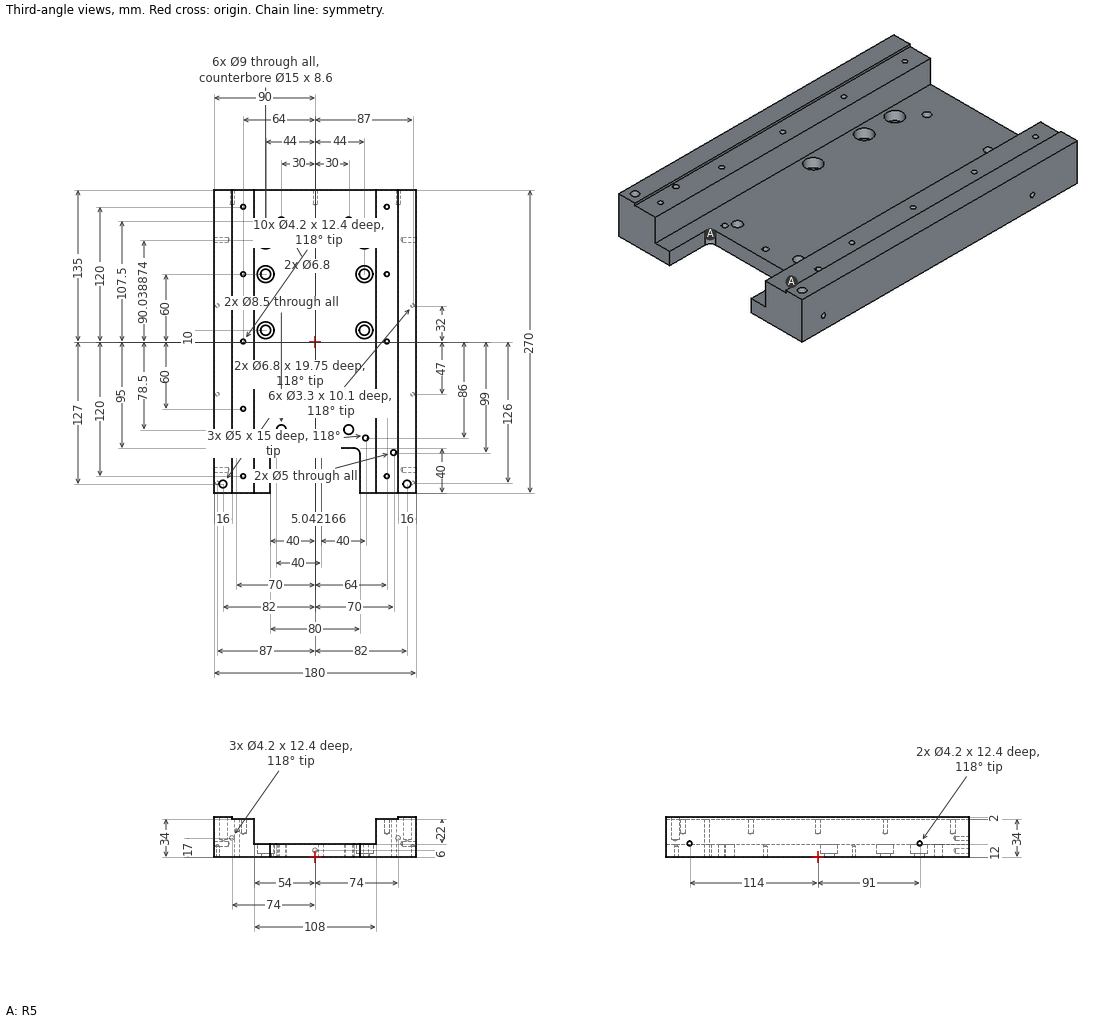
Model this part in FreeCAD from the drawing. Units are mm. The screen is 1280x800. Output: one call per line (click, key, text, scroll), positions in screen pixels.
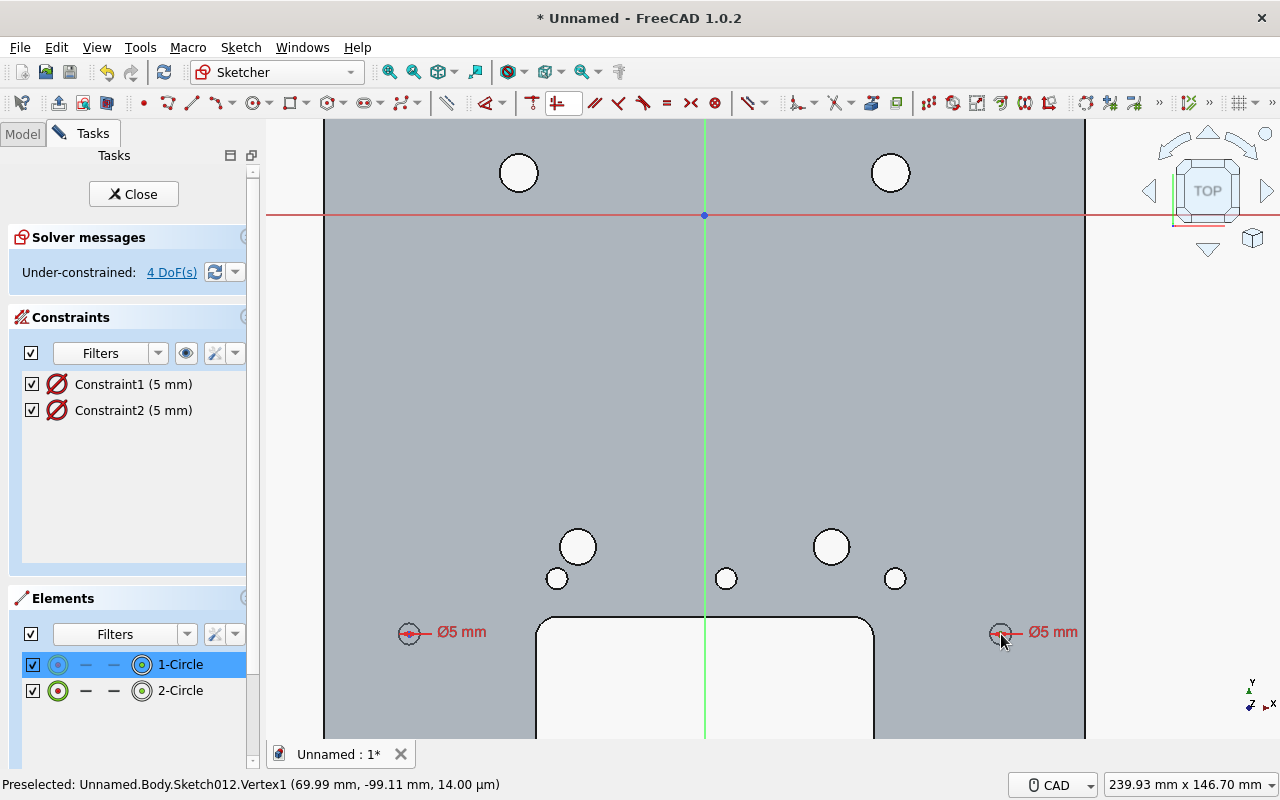
click(409, 634)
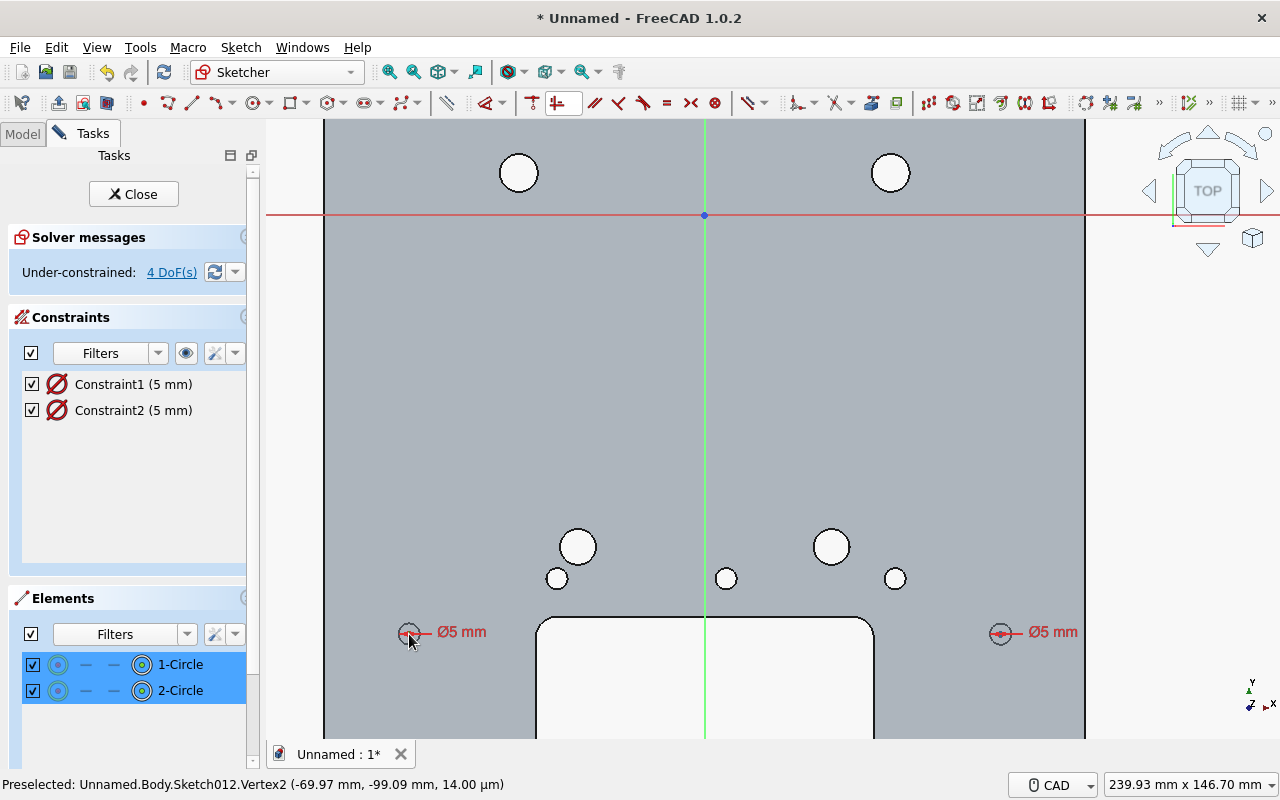
key(h)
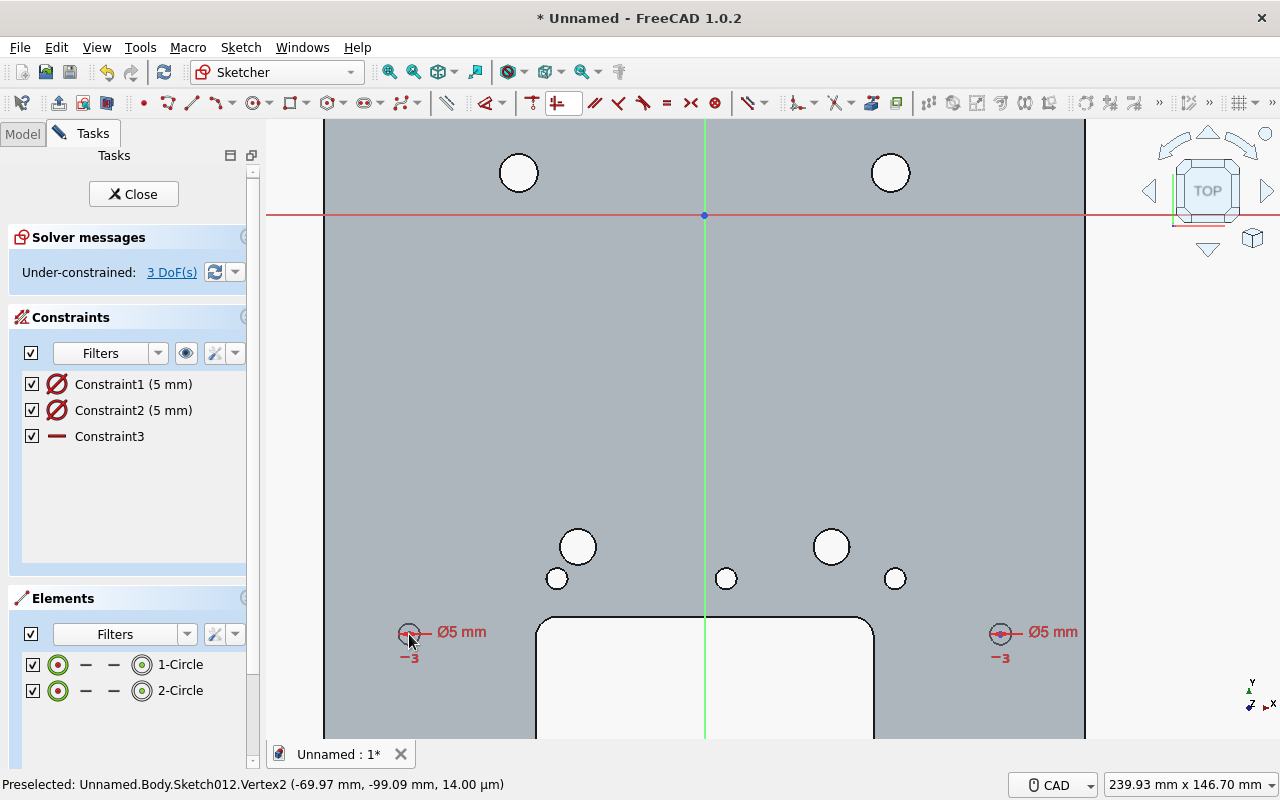
click(486, 104)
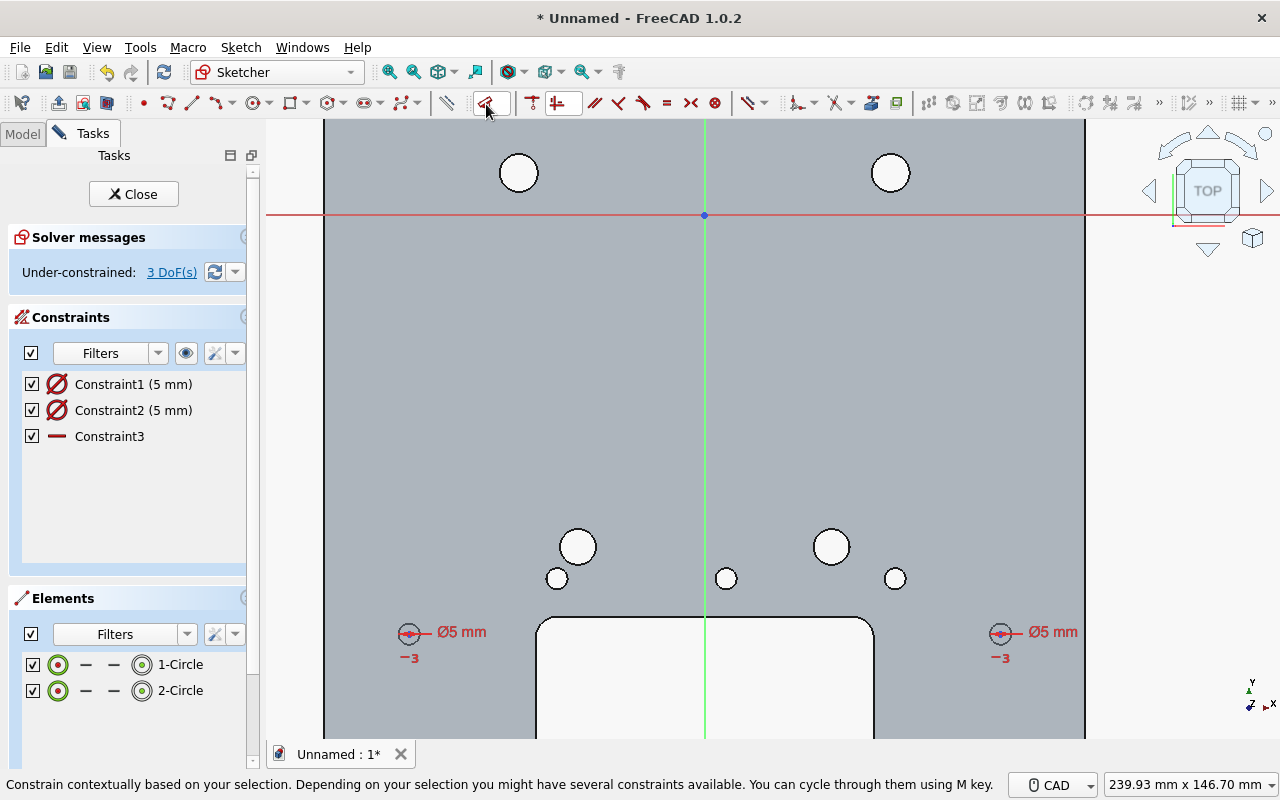
click(1001, 634)
click(853, 181)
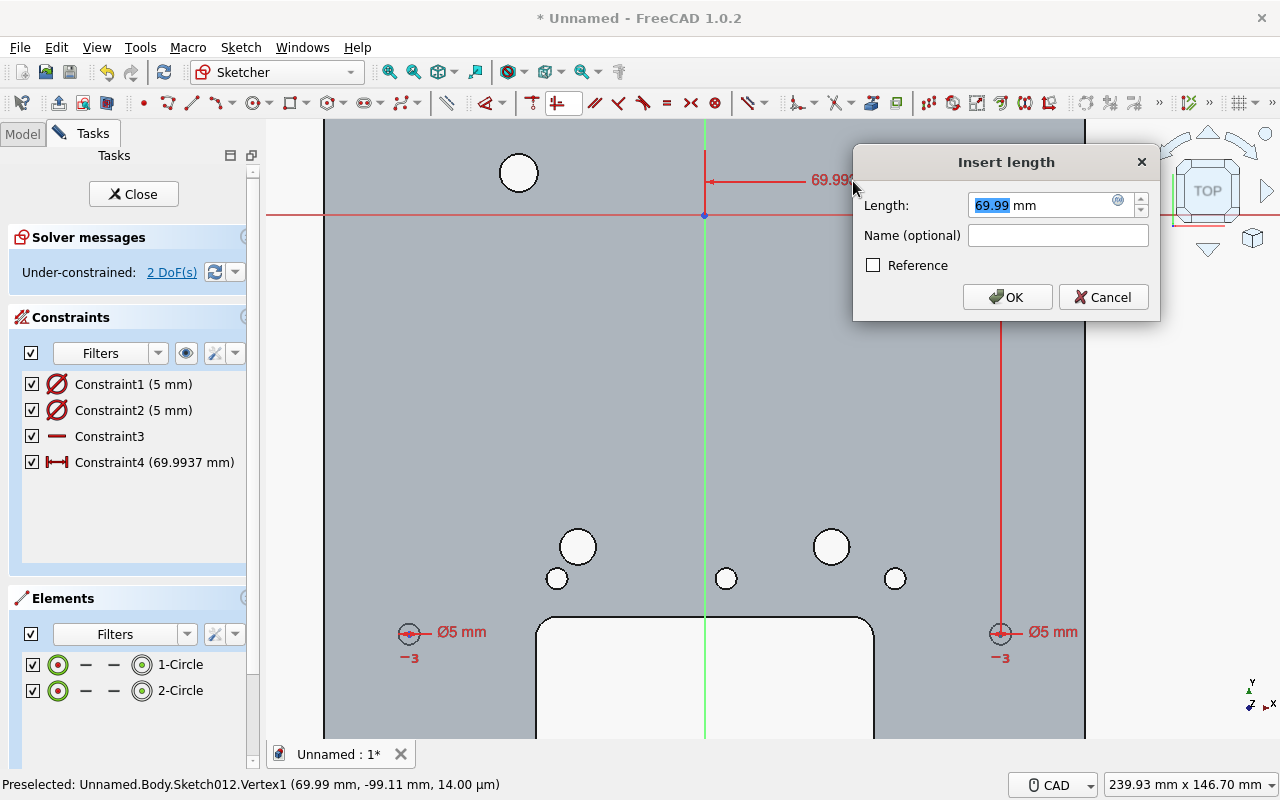
text(70)
key(Return)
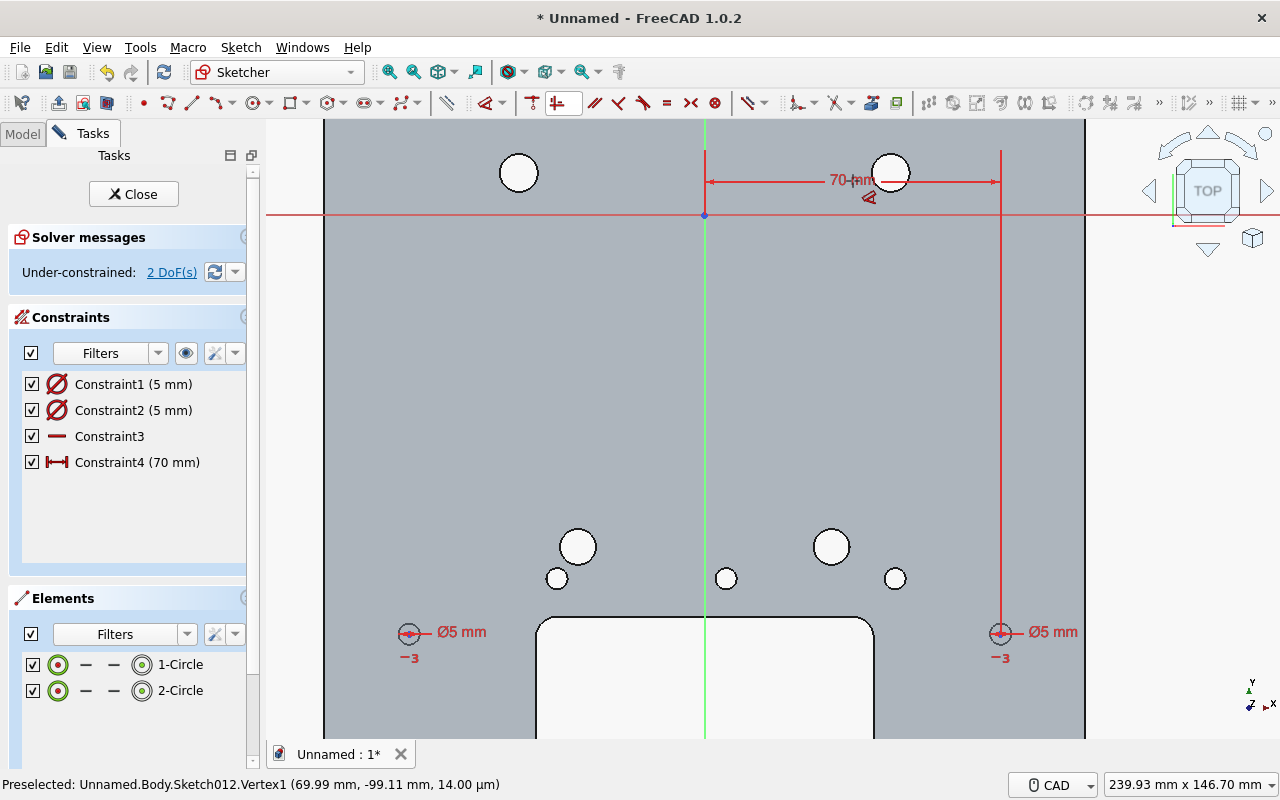
click(1001, 634)
click(1035, 425)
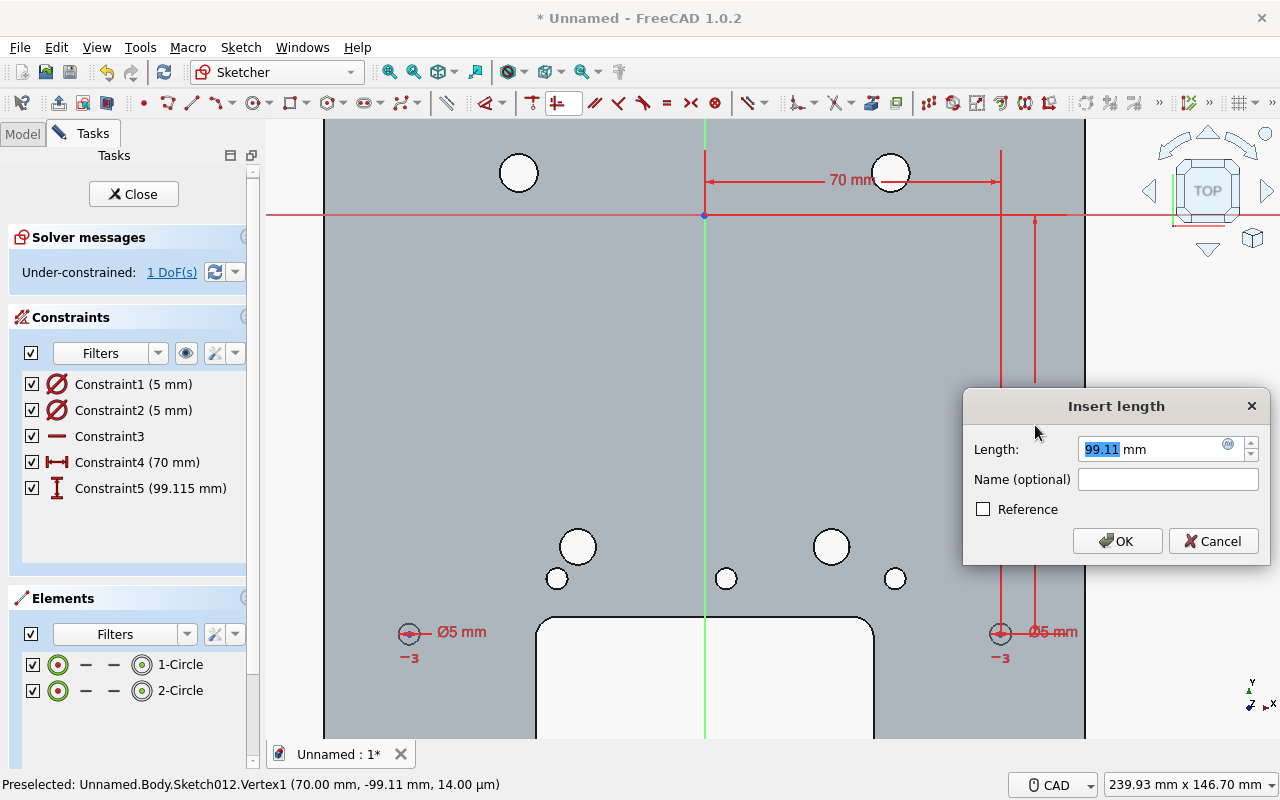
text(99)
key(Return)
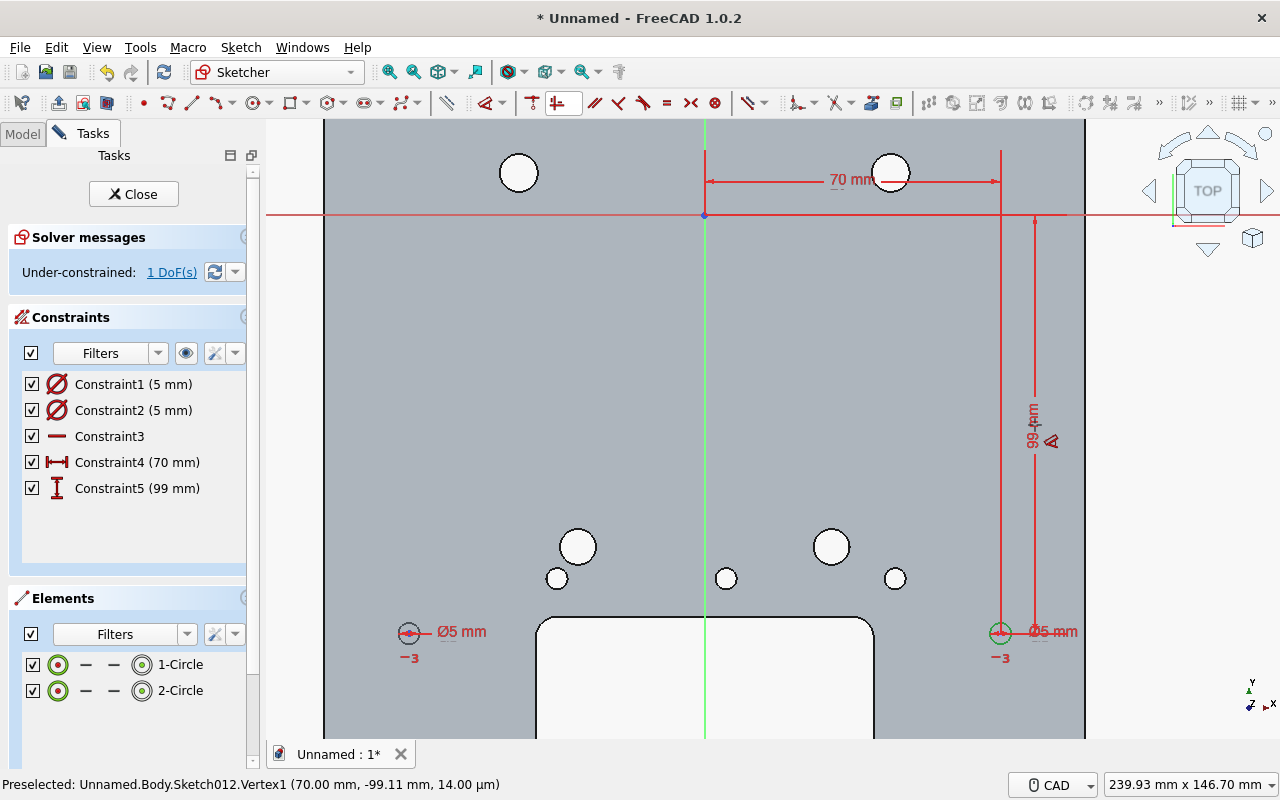
click(409, 634)
click(557, 181)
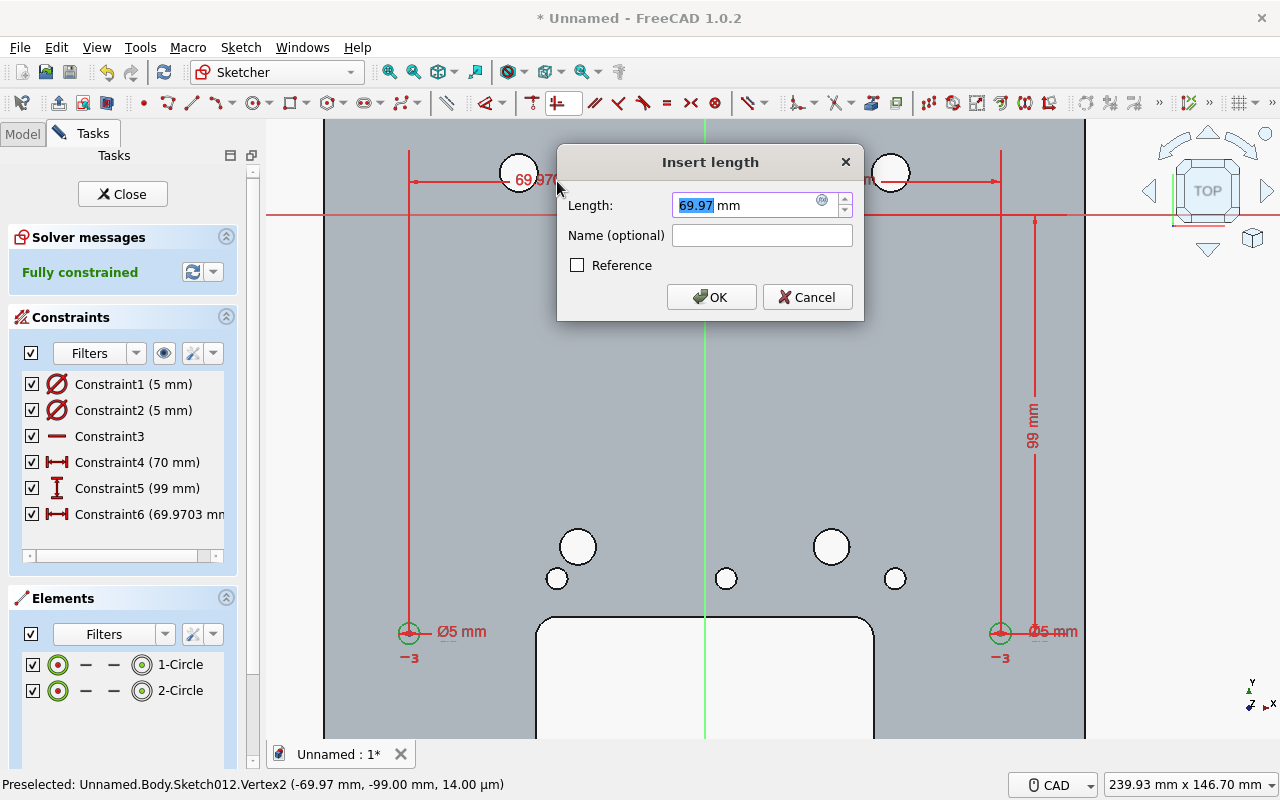
text(70)
key(Return)
key(Escape)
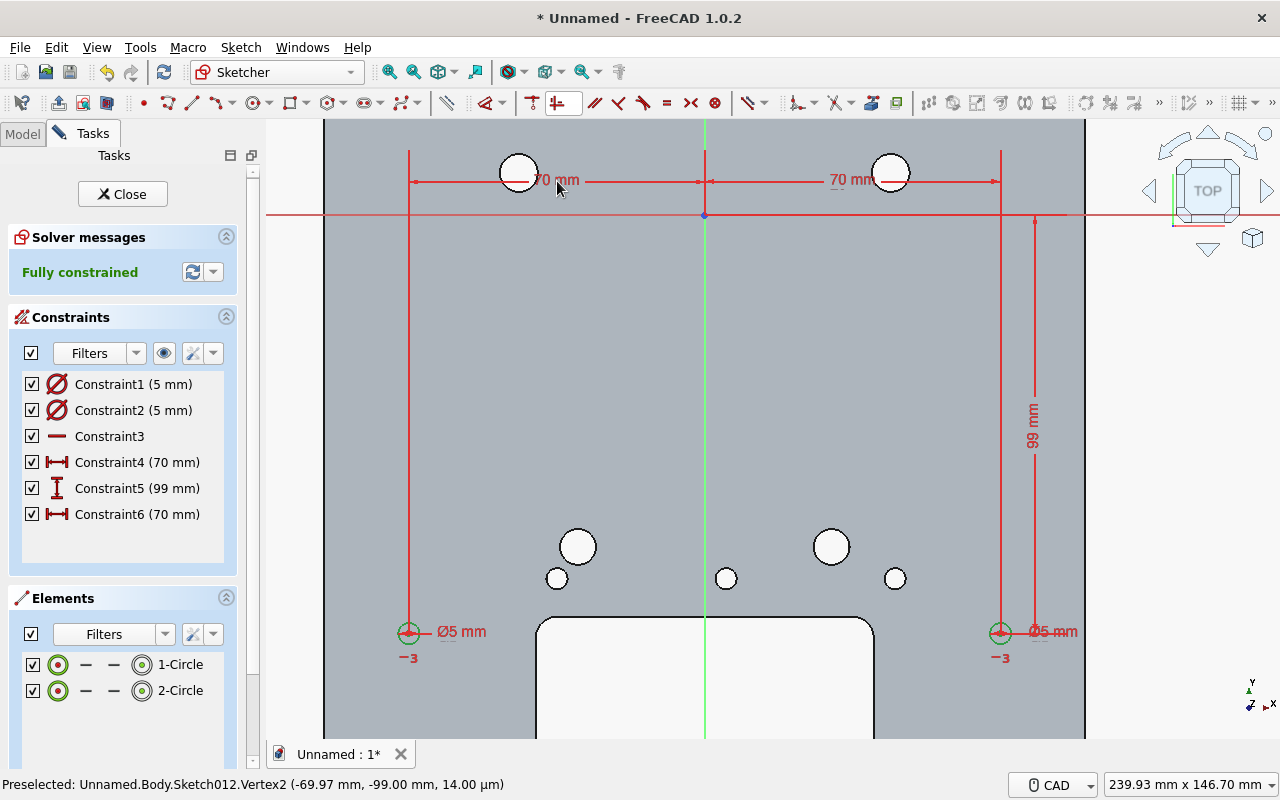
click(123, 194)